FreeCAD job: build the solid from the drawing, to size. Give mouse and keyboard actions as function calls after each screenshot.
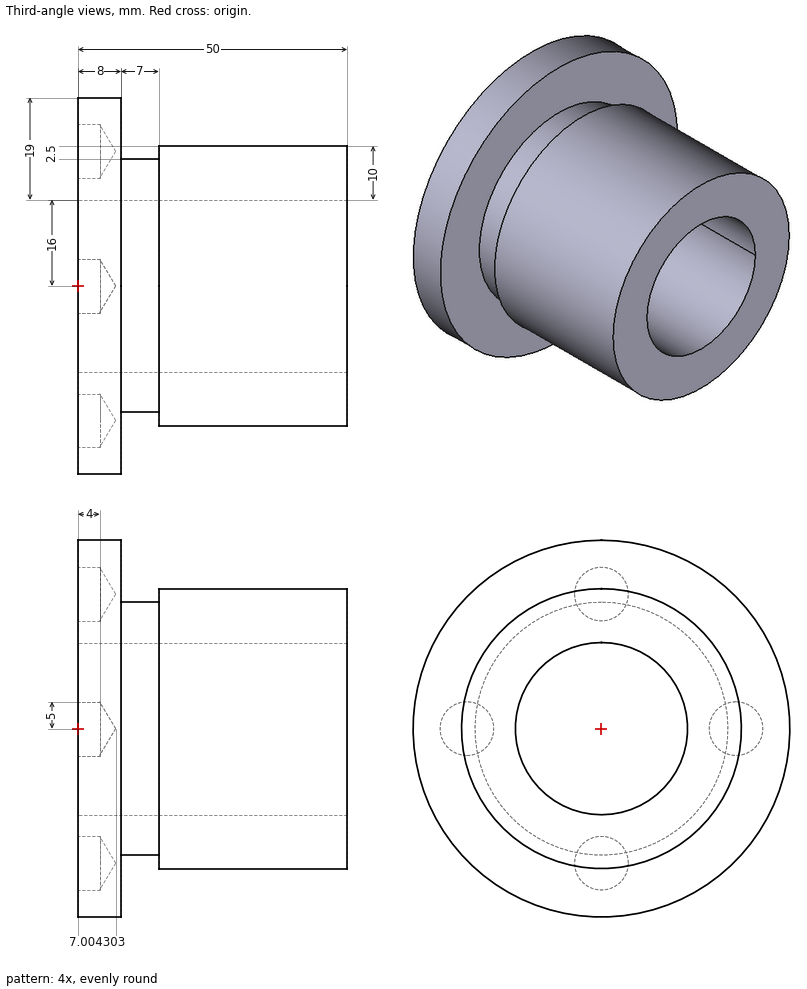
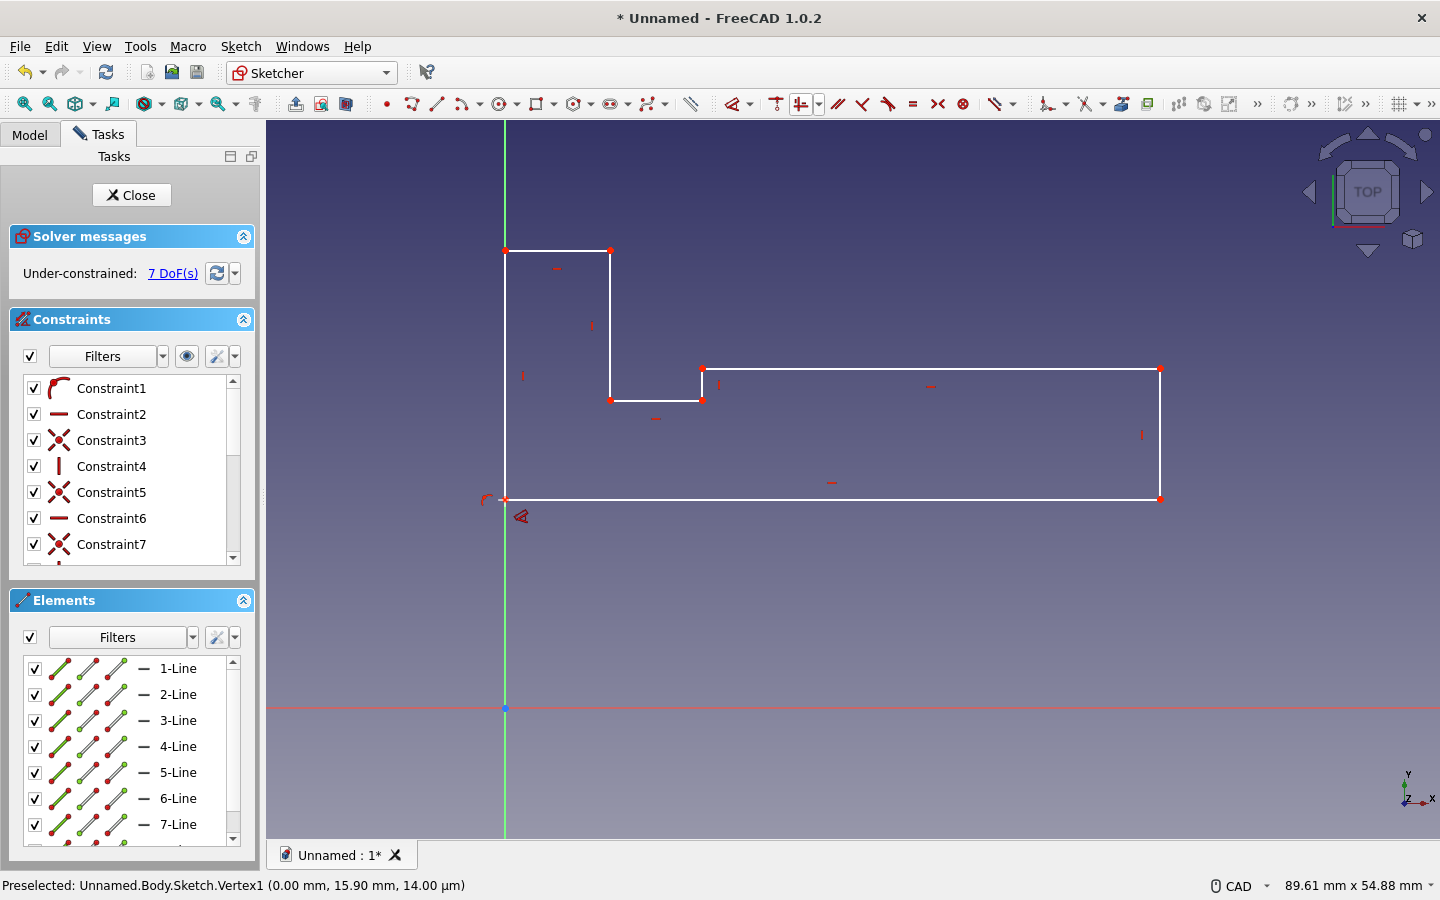
click(674, 401)
click(656, 367)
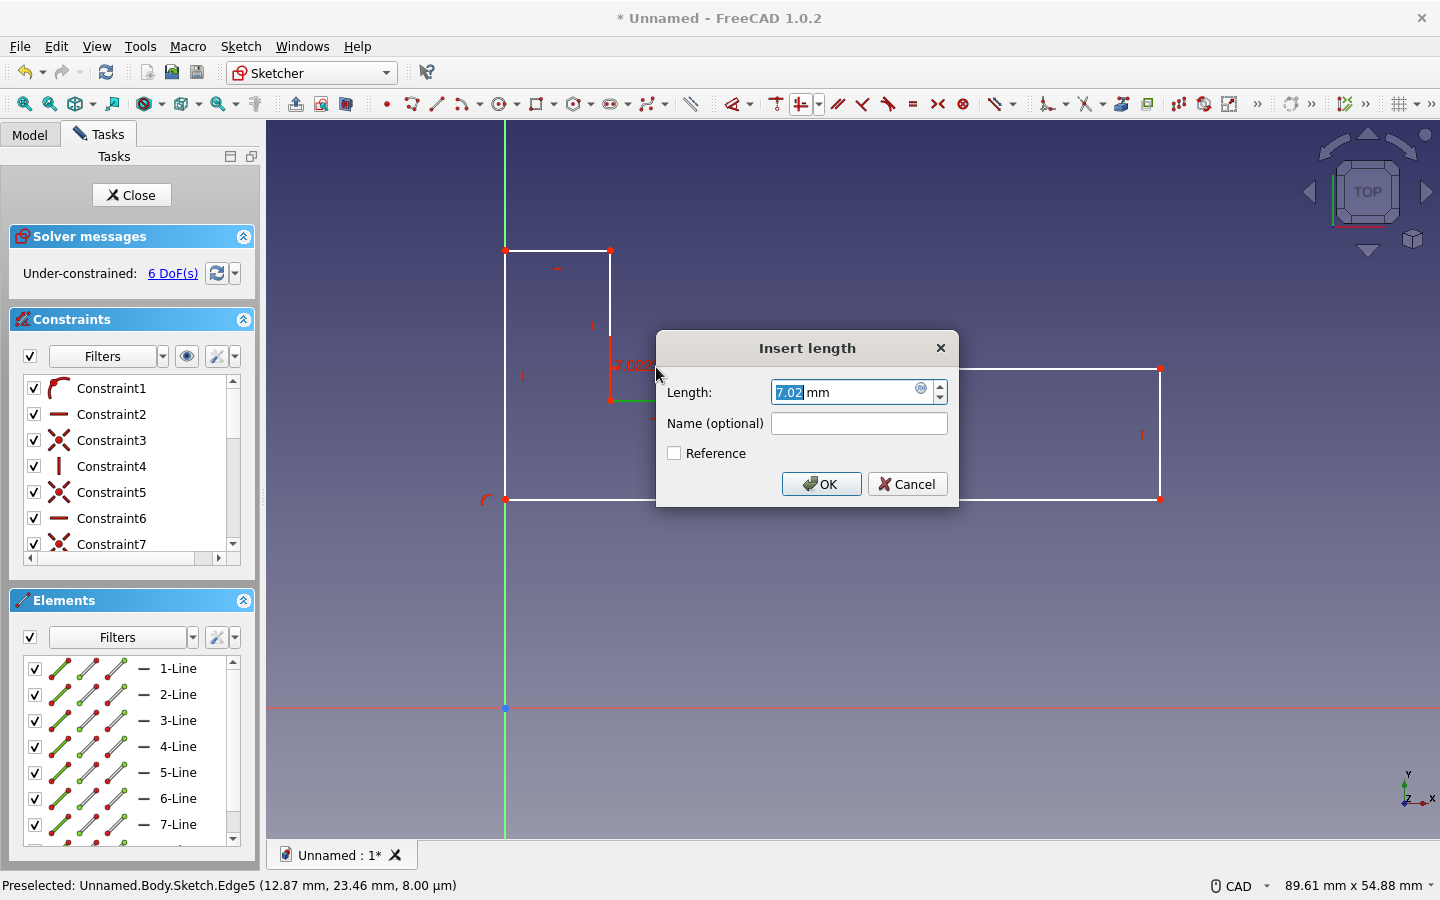
text(7)
key(Return)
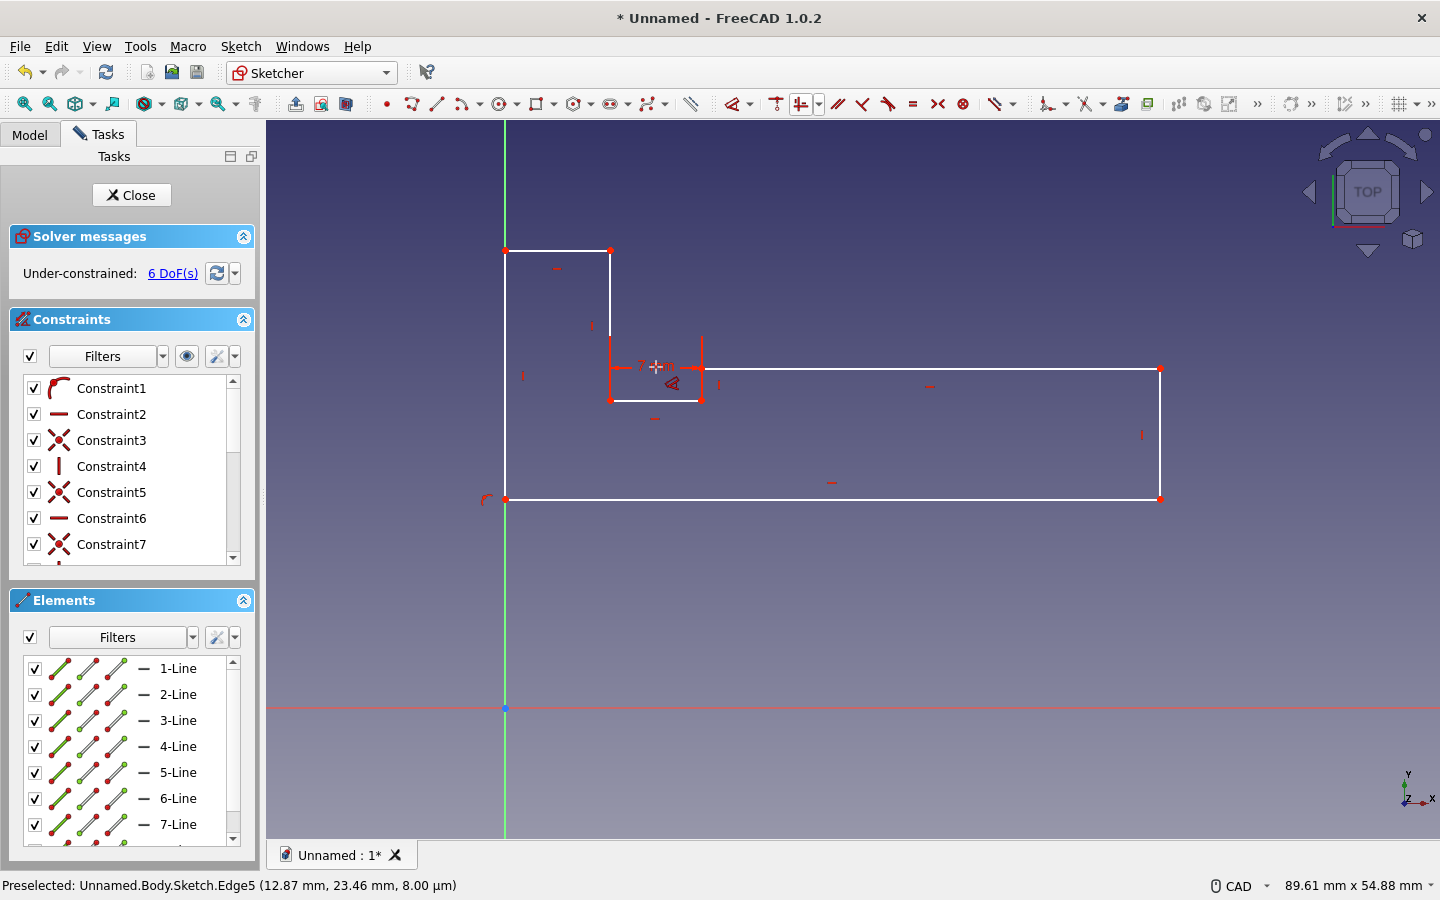
click(579, 251)
click(558, 217)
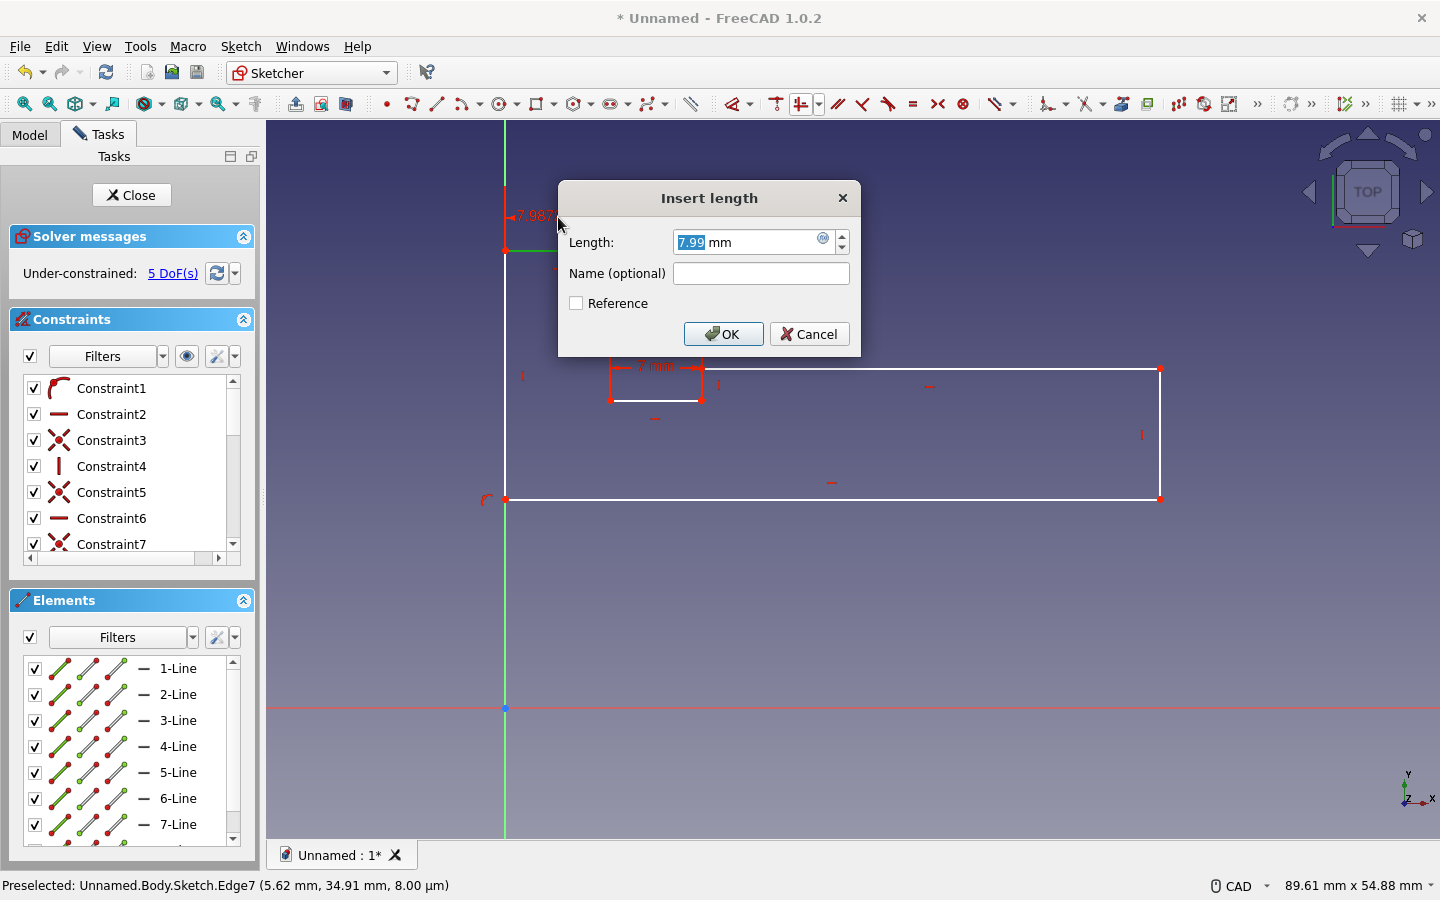
text(8)
key(Return)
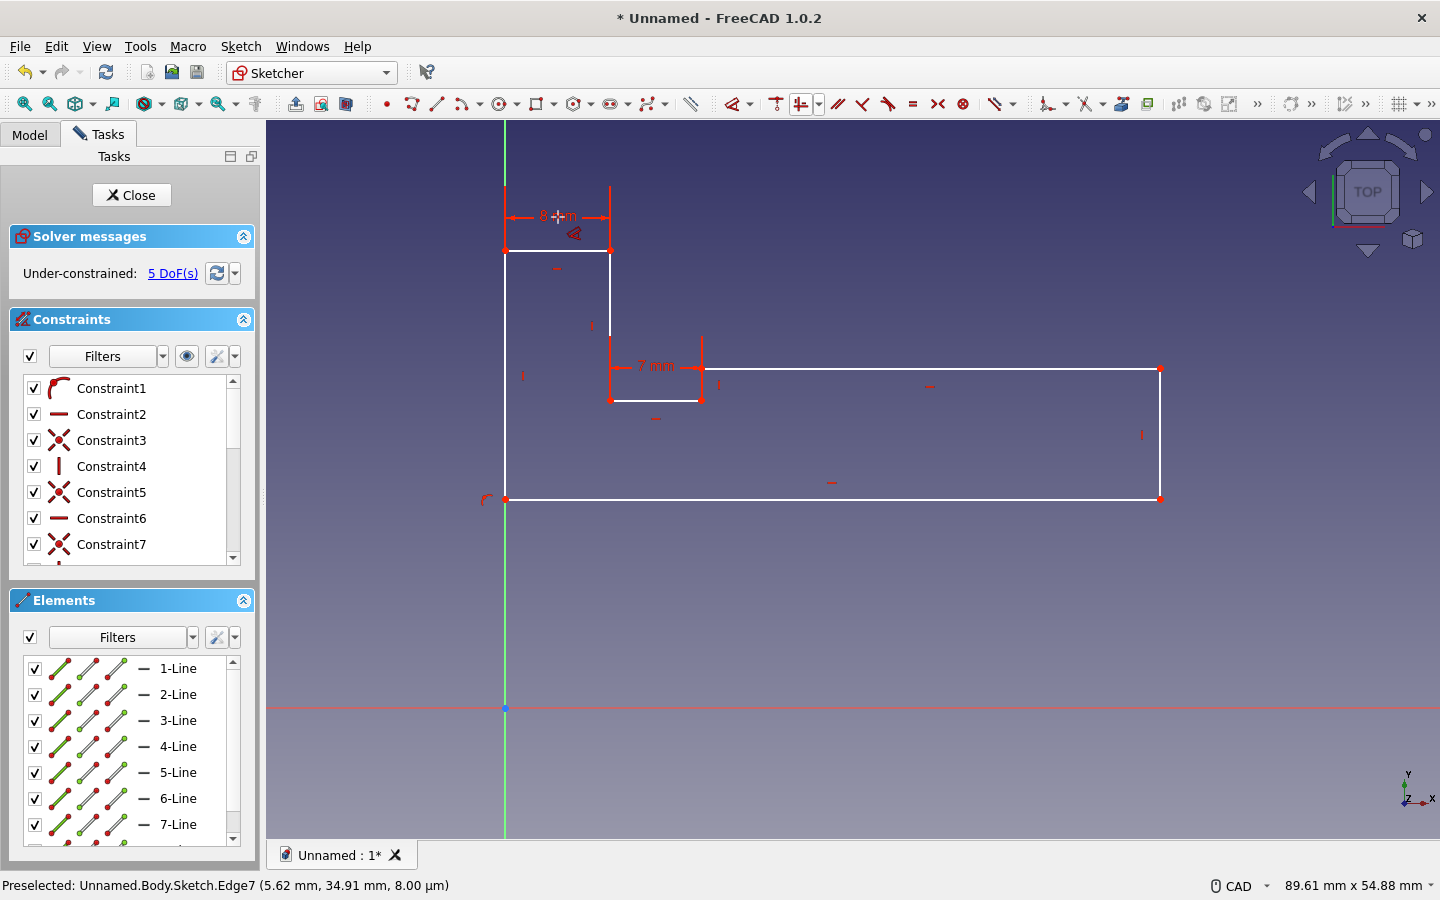
click(702, 500)
click(833, 534)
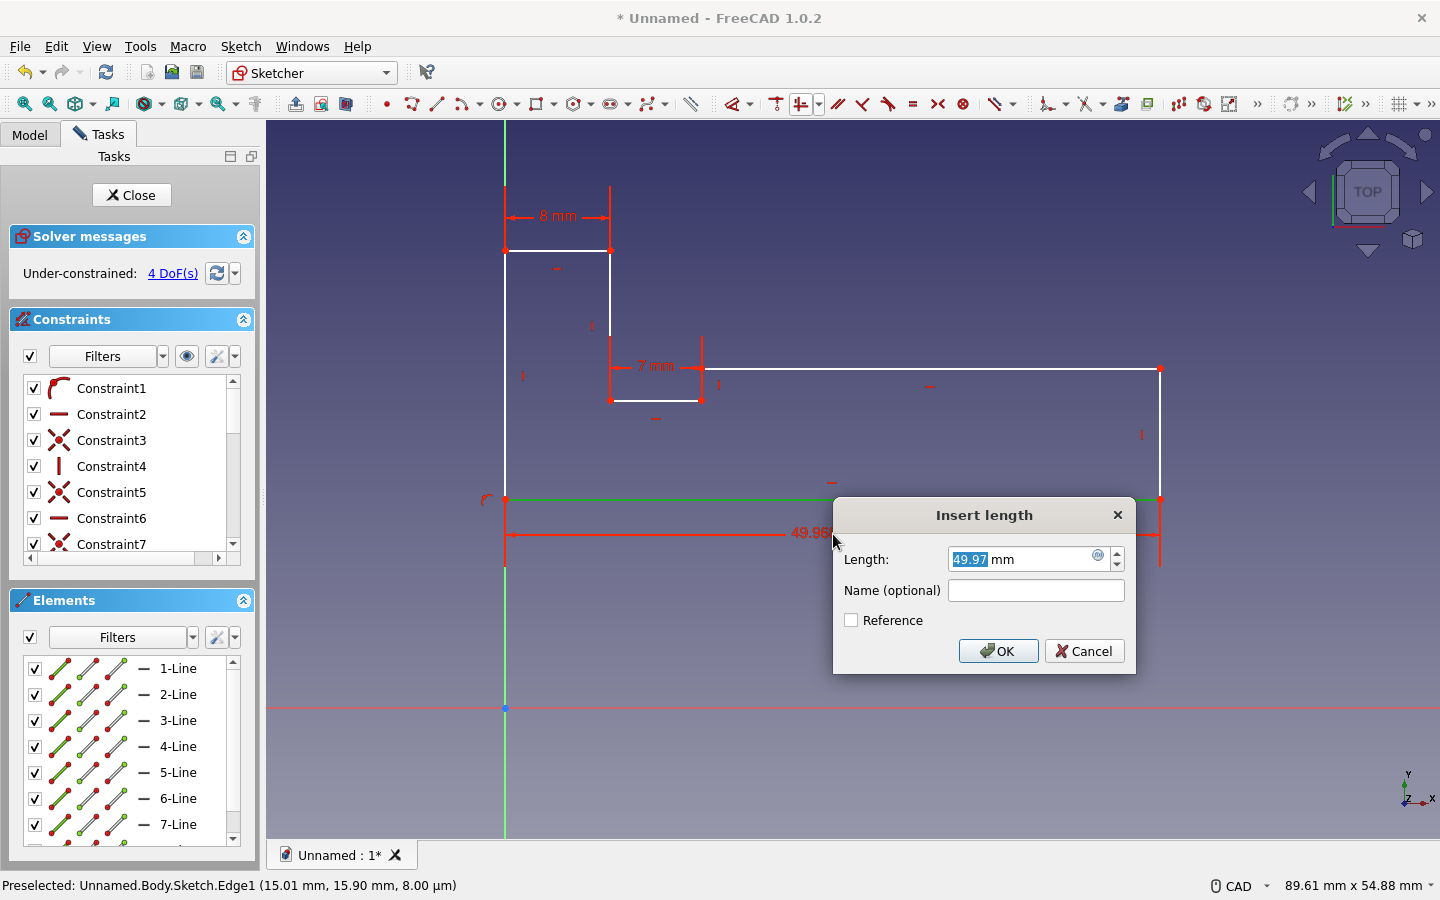
text(50)
key(Return)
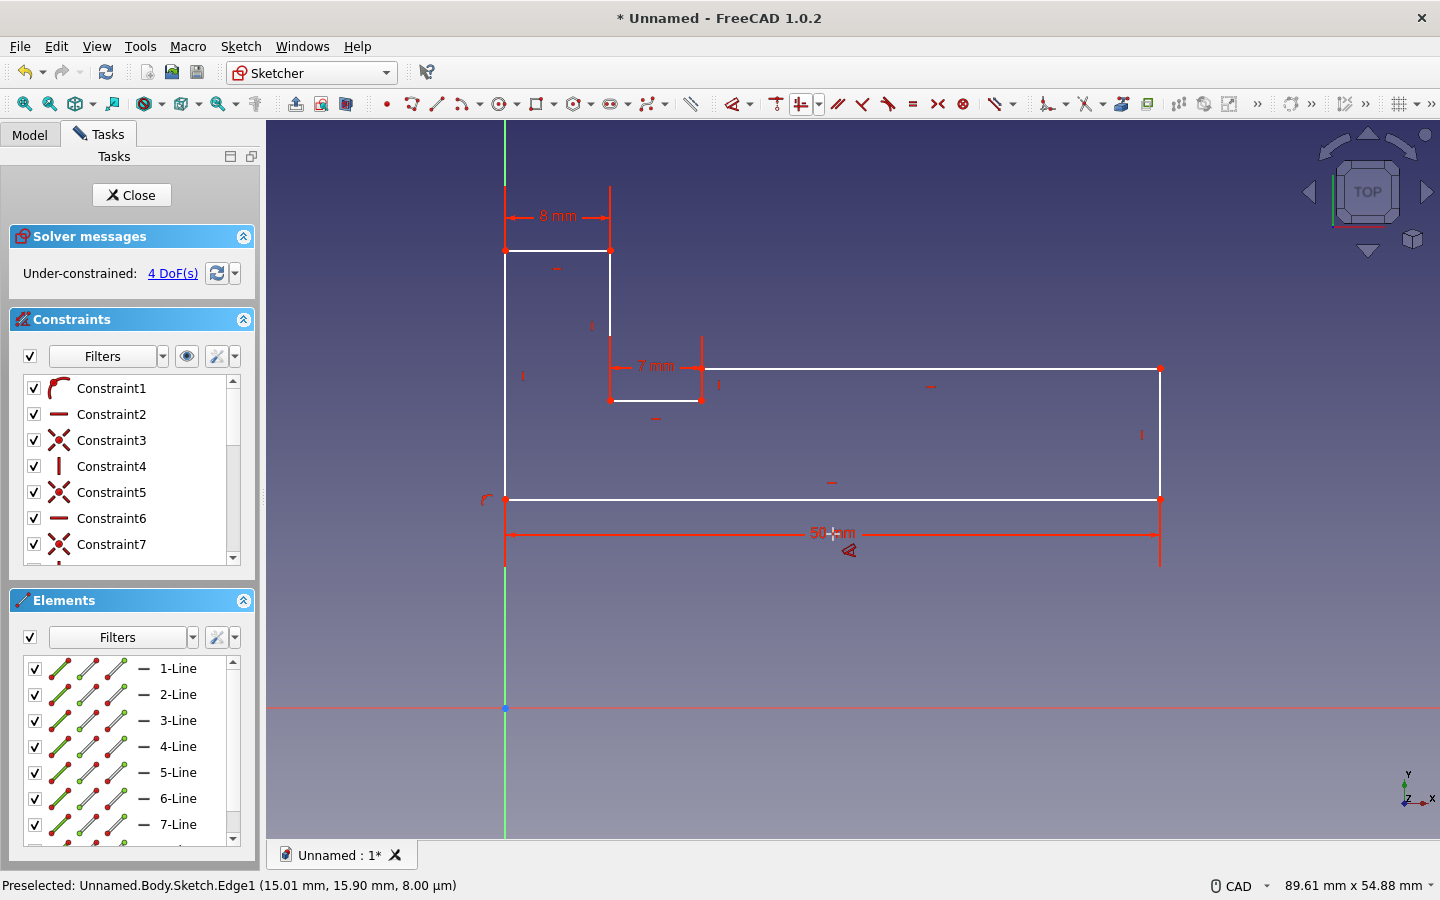
click(1160, 461)
click(1194, 434)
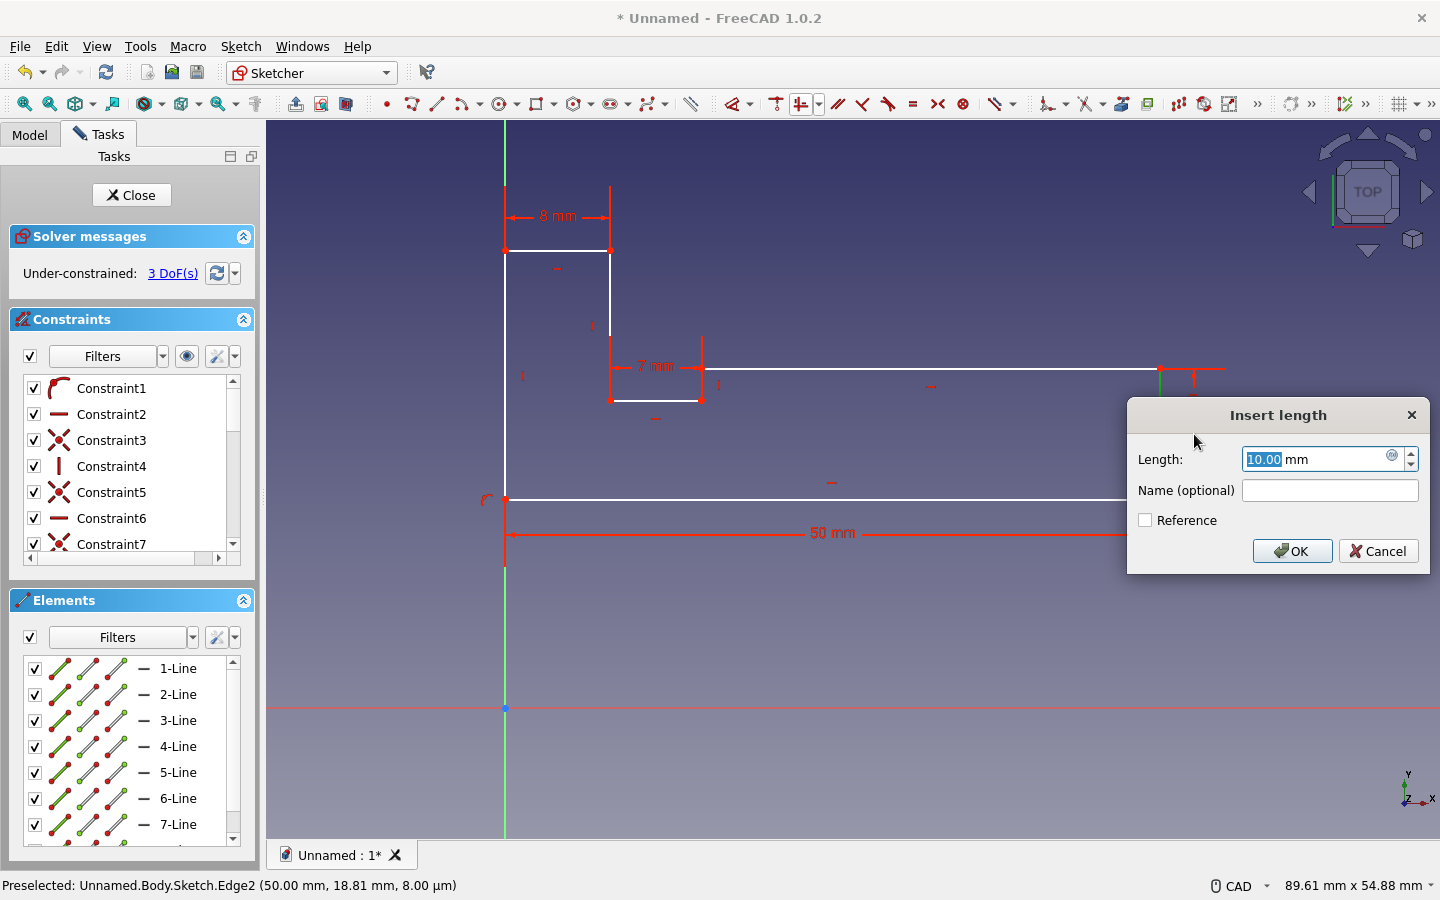
text(10)
key(Return)